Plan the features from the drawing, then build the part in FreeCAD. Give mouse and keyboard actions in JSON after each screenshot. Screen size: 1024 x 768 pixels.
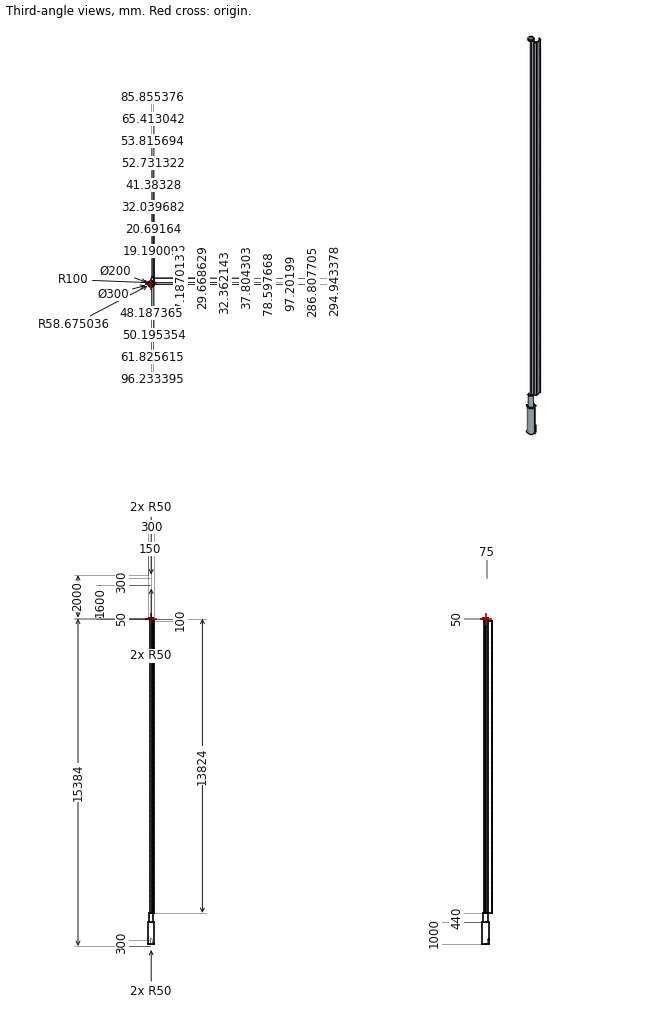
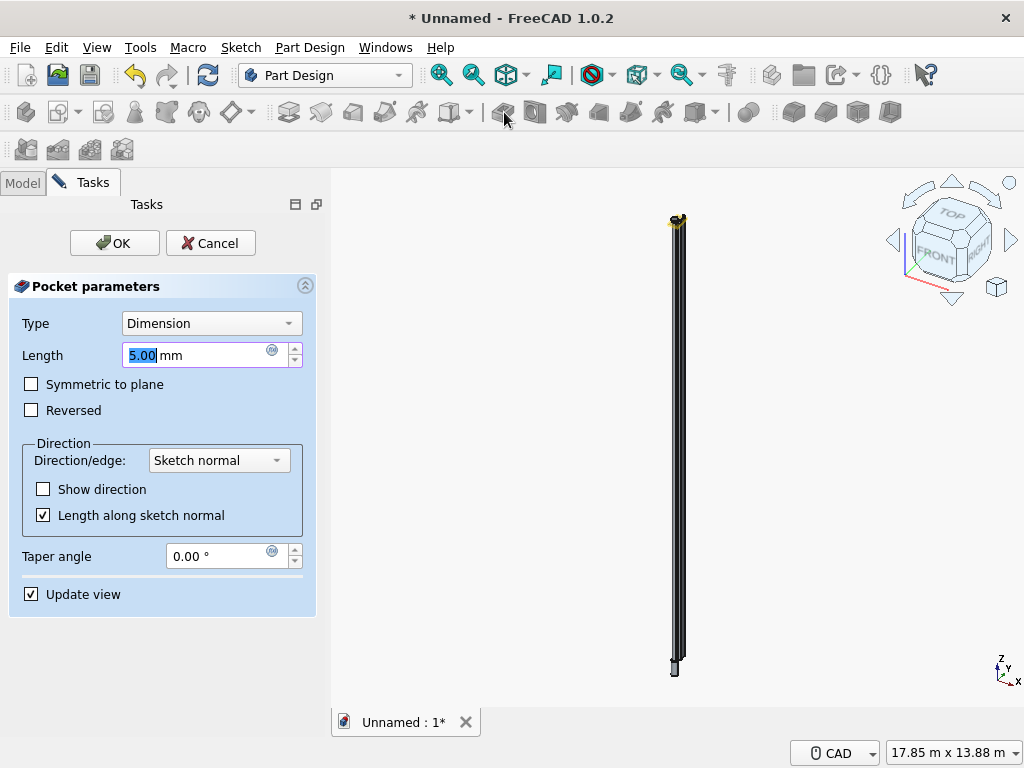
{"action": "type", "text": "100"}
{"action": "key", "text": "Tab"}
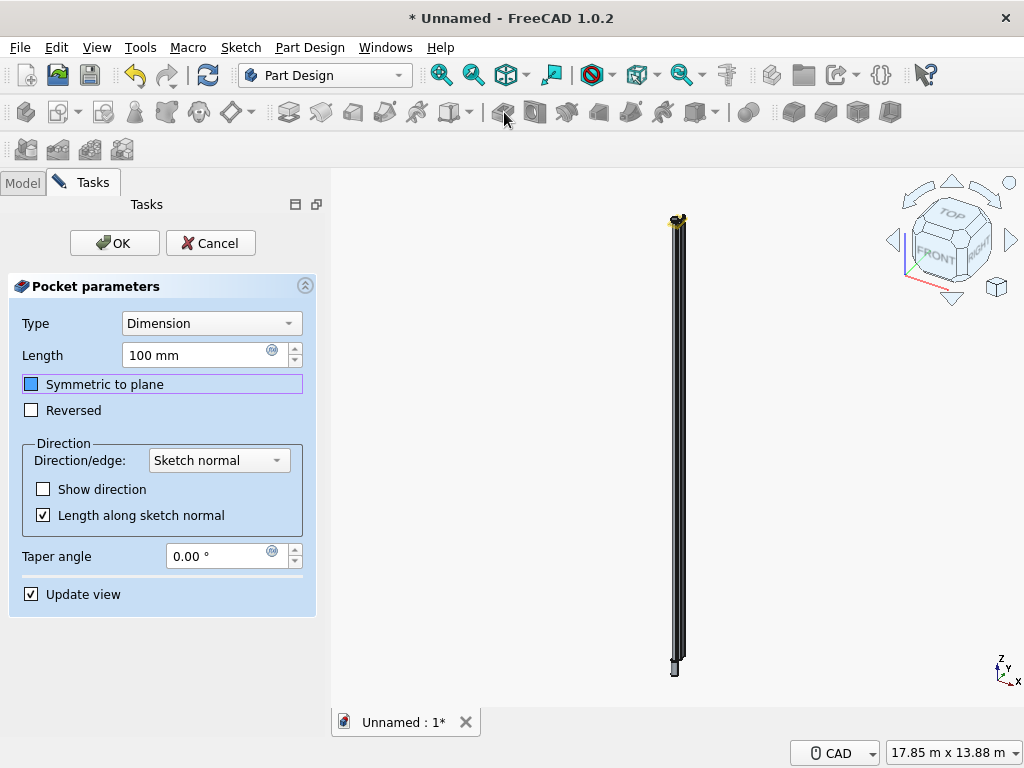
{"action": "left_click", "coordinate": [30, 410]}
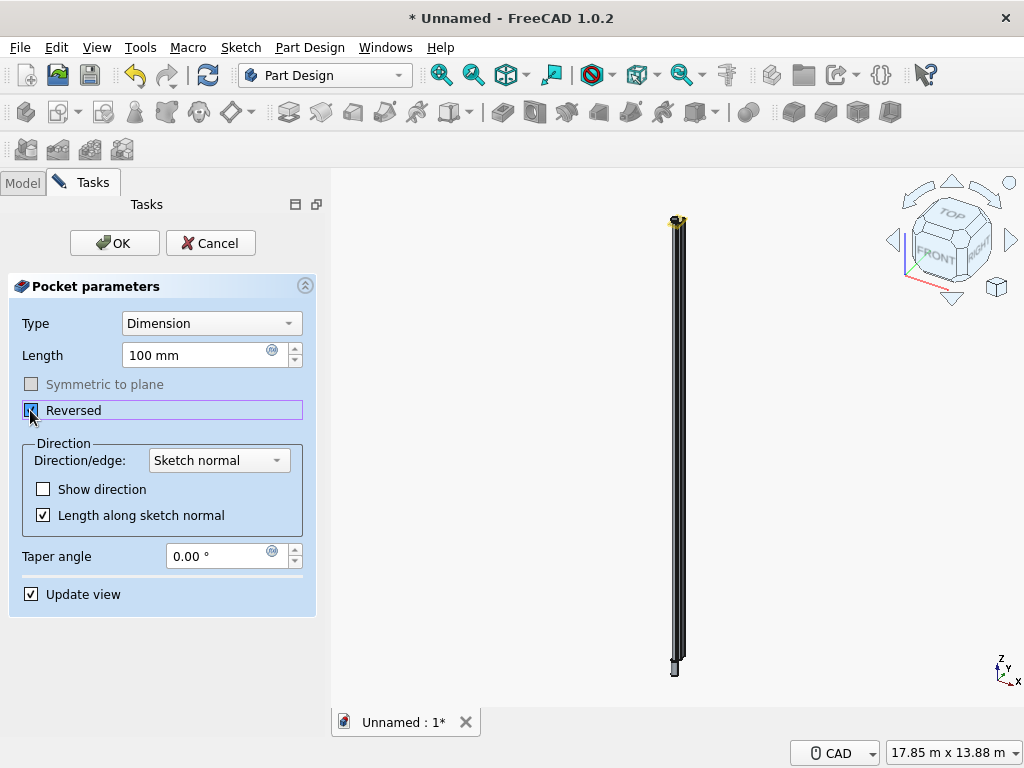
{"action": "left_click", "coordinate": [115, 243]}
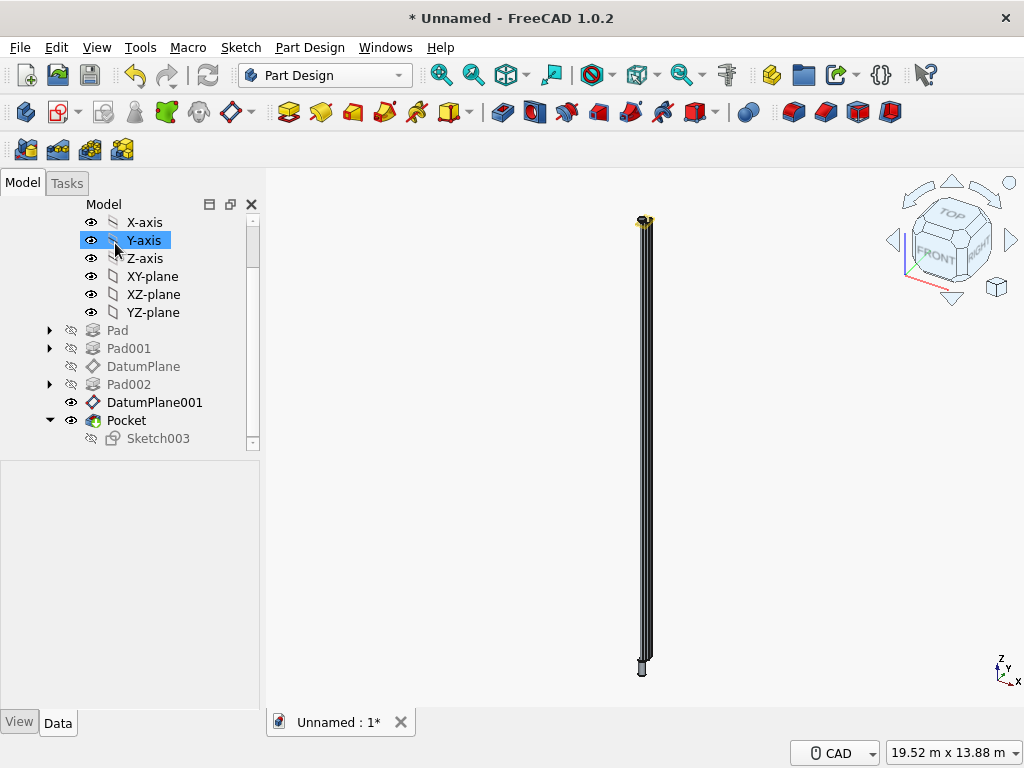
{"action": "left_click", "coordinate": [116, 402]}
{"action": "key", "text": "space"}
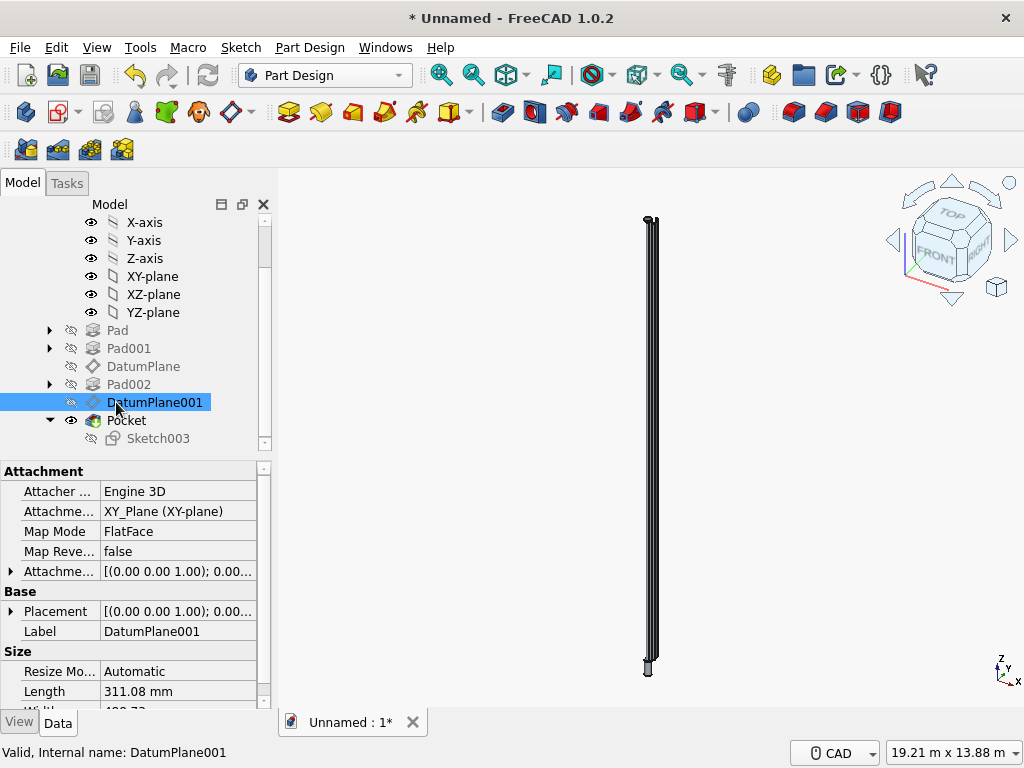
{"action": "scroll", "coordinate": [648, 218], "scroll_direction": "up", "scroll_amount": 6}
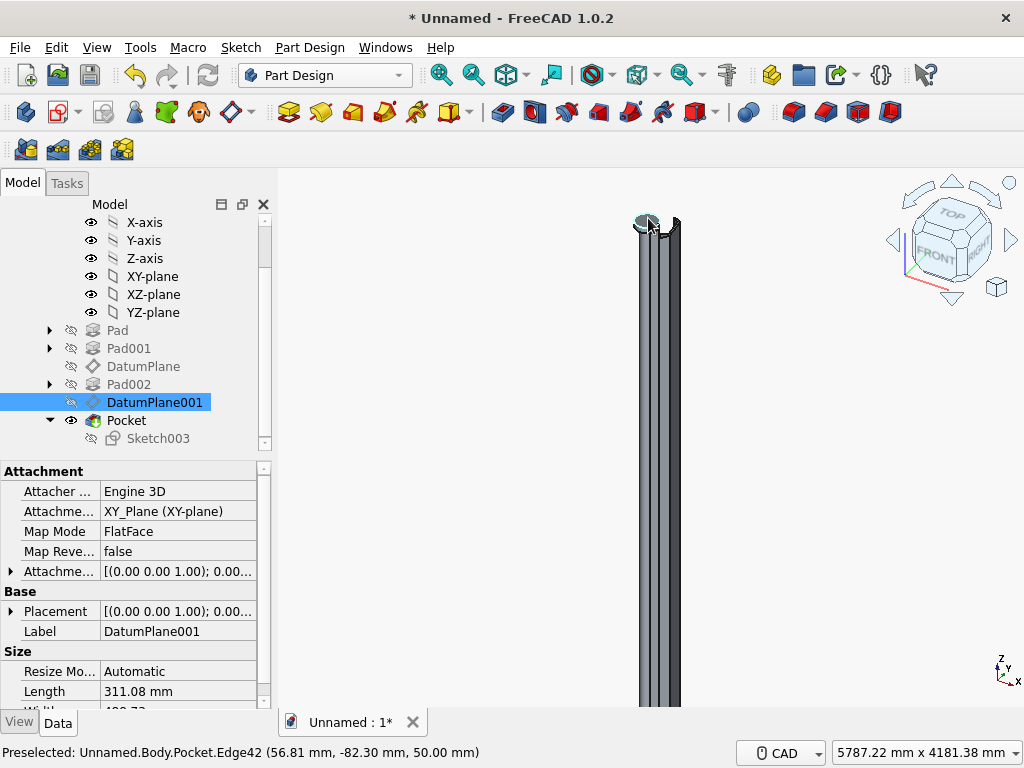
{"action": "left_click", "coordinate": [649, 218]}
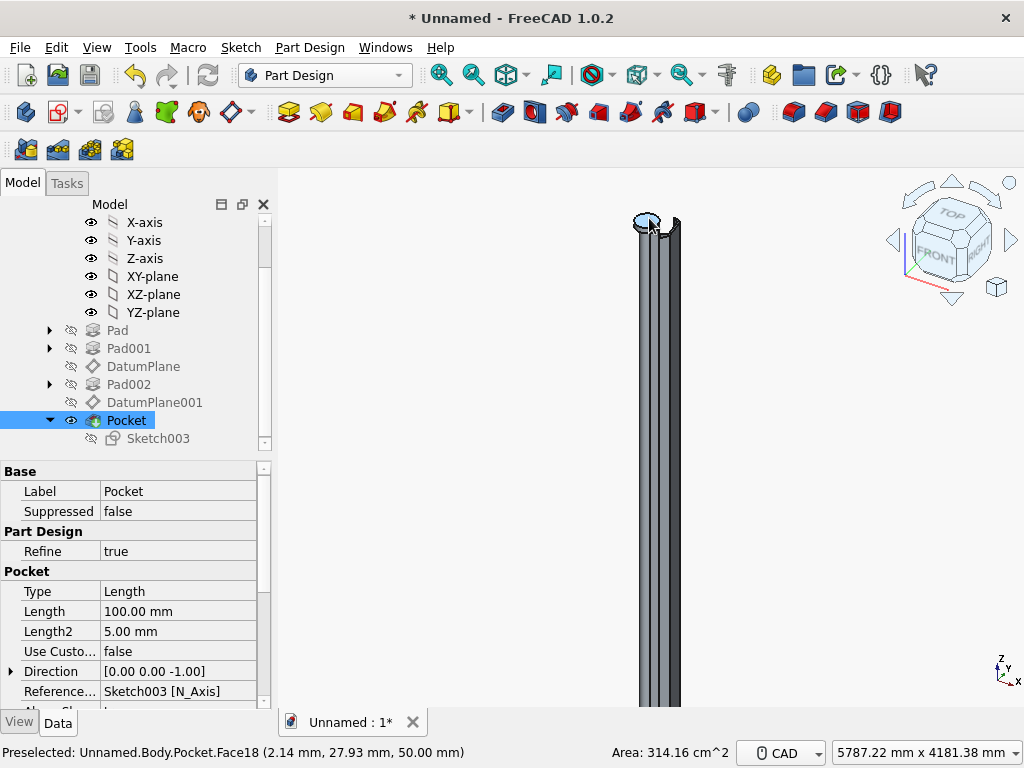
{"action": "left_click", "coordinate": [58, 112]}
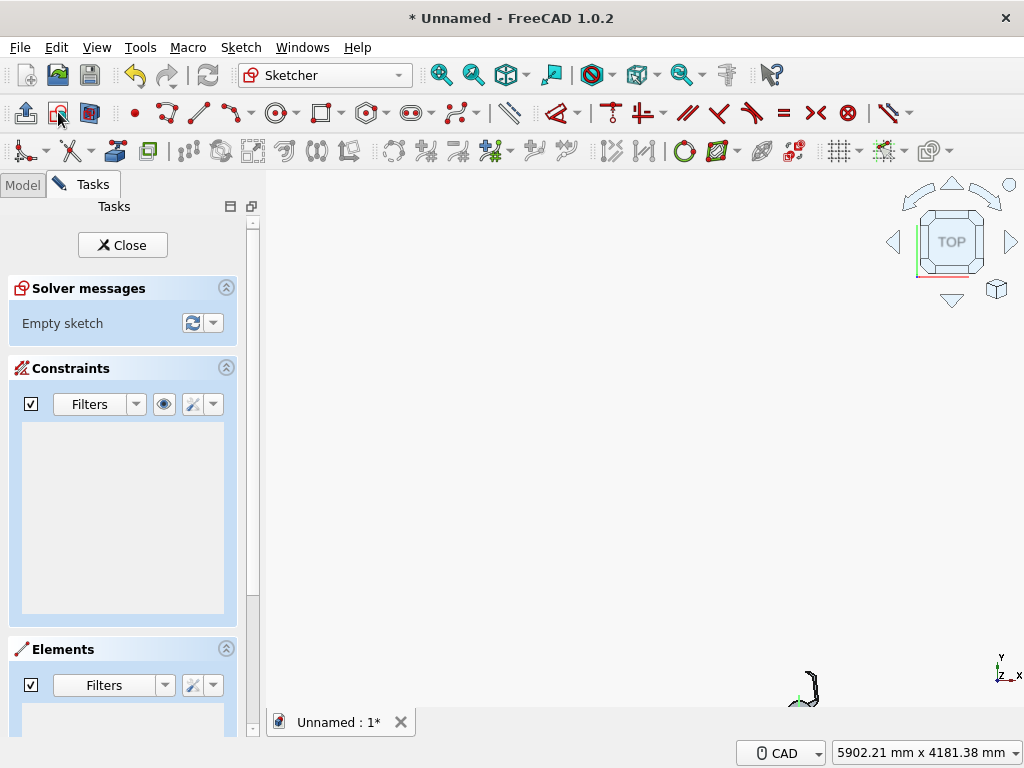
{"action": "scroll", "coordinate": [576, 438], "scroll_direction": "down", "scroll_amount": 5}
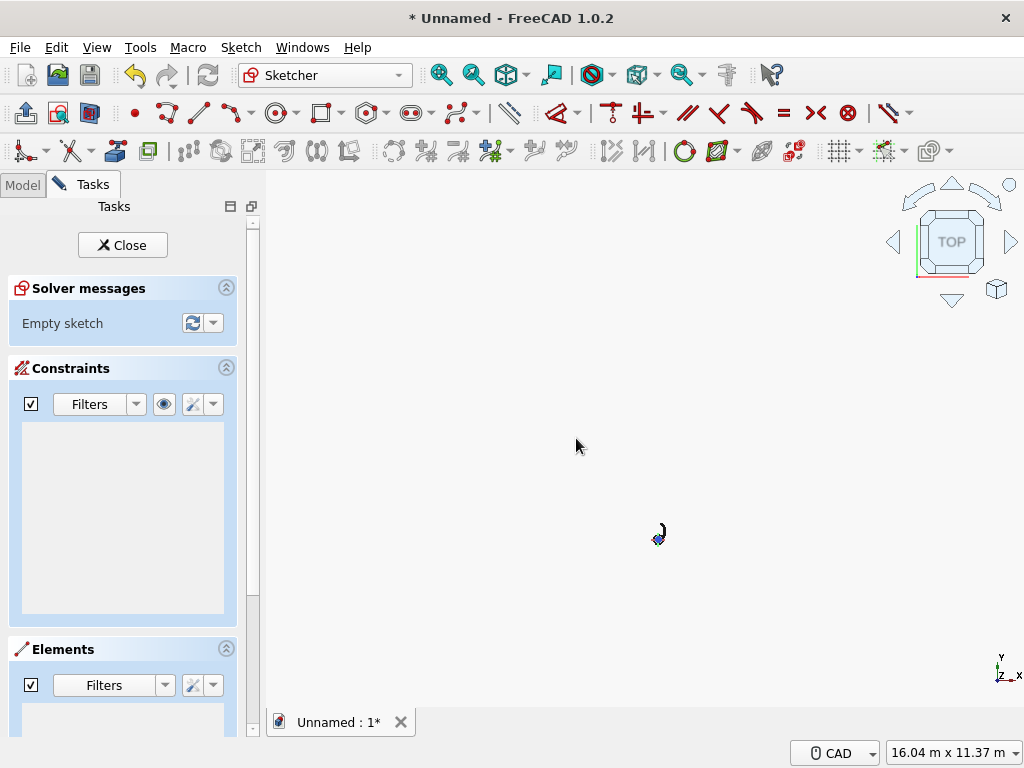
{"action": "scroll", "coordinate": [663, 545], "scroll_direction": "up", "scroll_amount": 15}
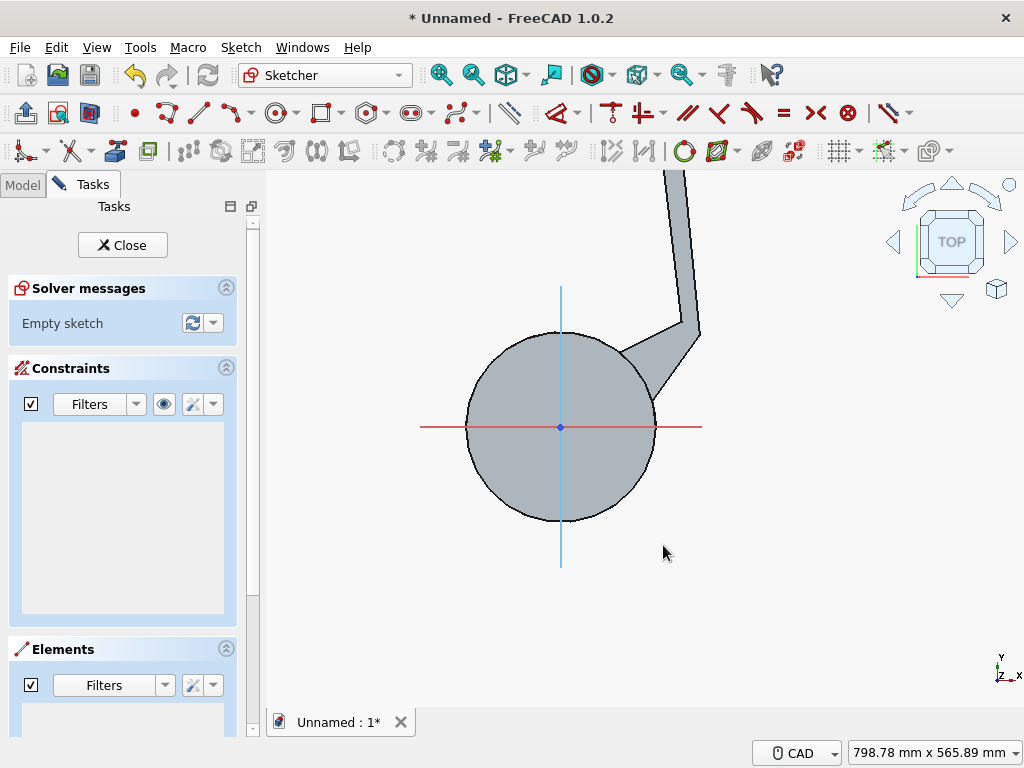
{"action": "left_click", "coordinate": [276, 114]}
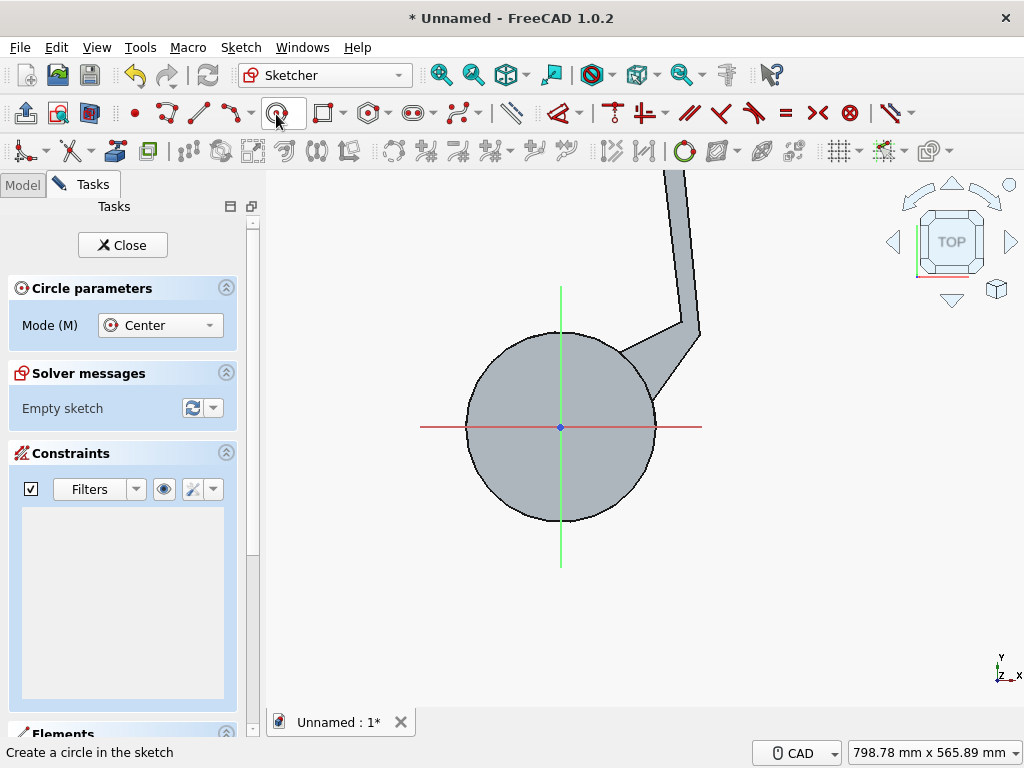
{"action": "left_click", "coordinate": [561, 427]}
{"action": "left_click", "coordinate": [662, 326]}
{"action": "key", "text": "Escape"}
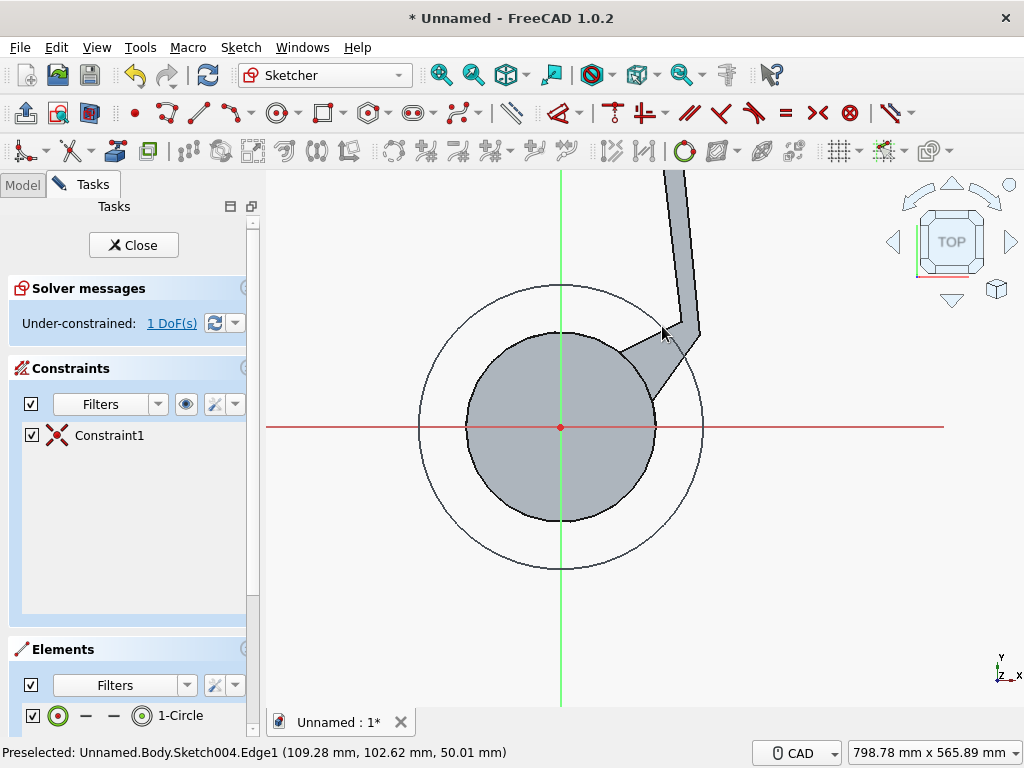
{"action": "left_click", "coordinate": [558, 114]}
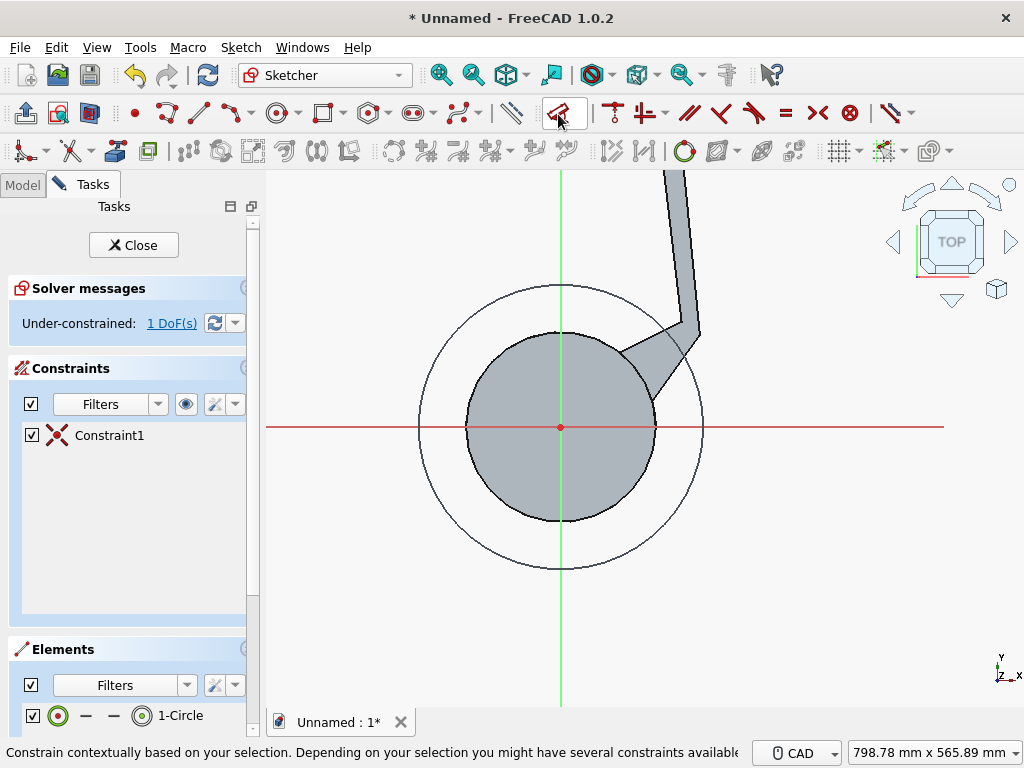
{"action": "left_click", "coordinate": [661, 326]}
{"action": "left_click", "coordinate": [684, 303]}